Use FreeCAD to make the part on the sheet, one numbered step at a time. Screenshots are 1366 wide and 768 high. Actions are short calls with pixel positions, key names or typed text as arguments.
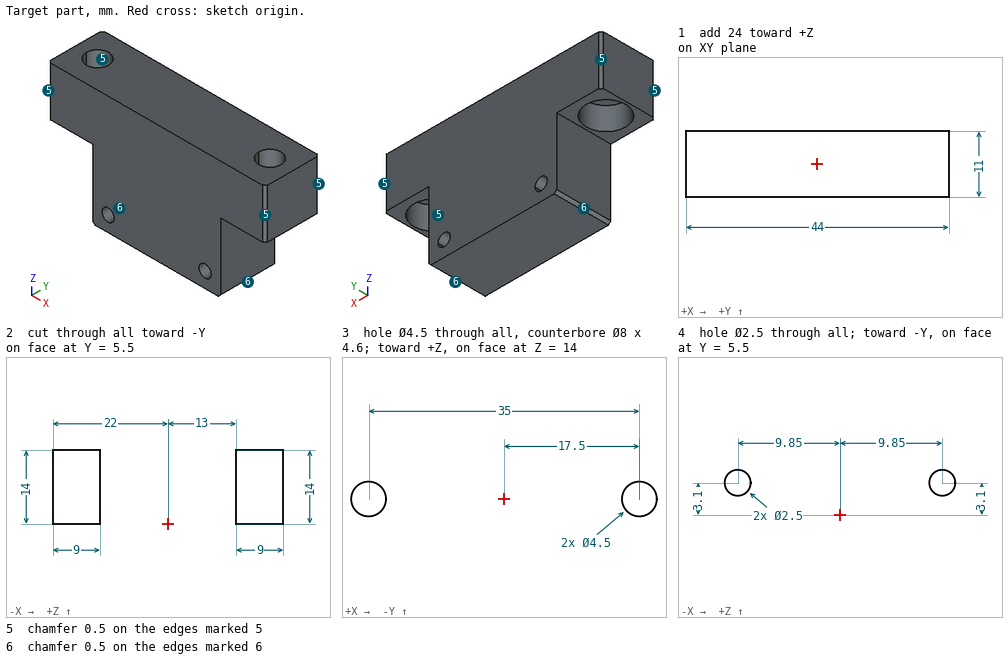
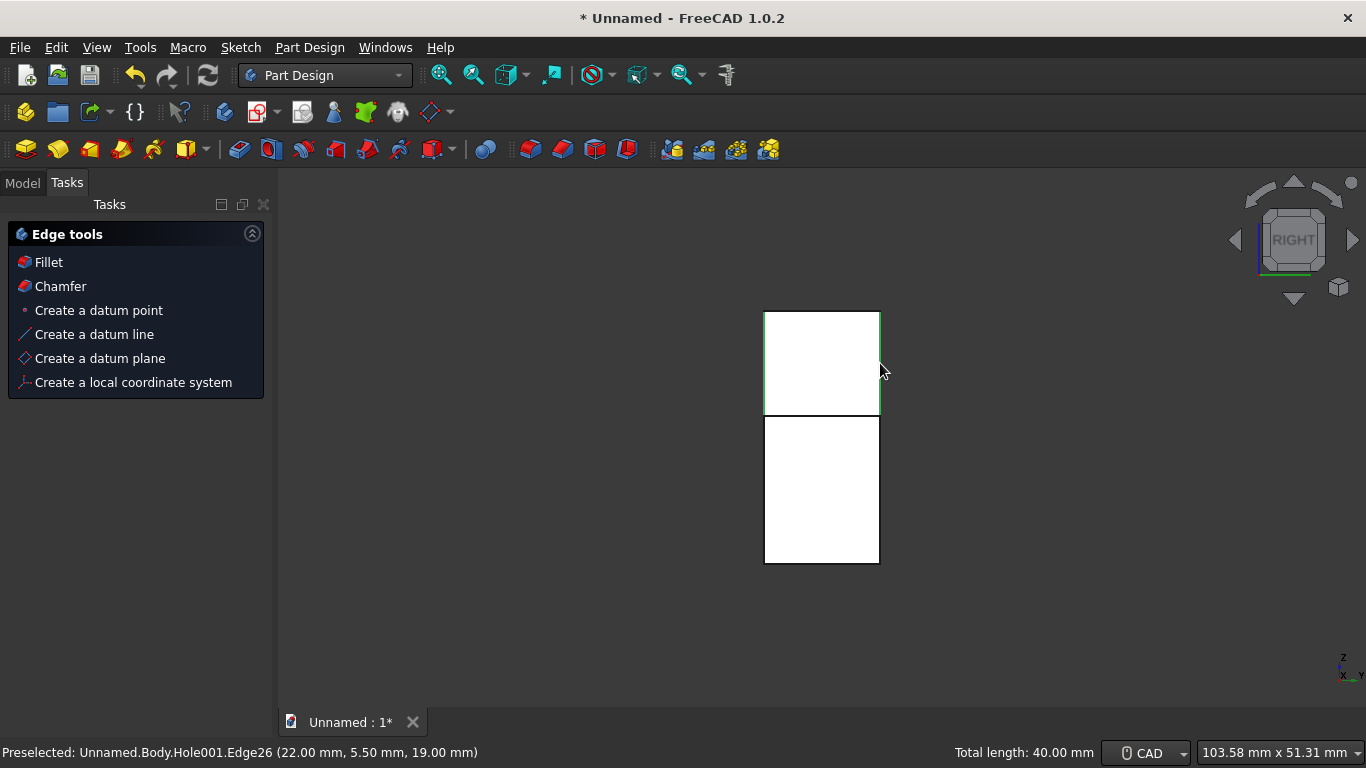
click(564, 150)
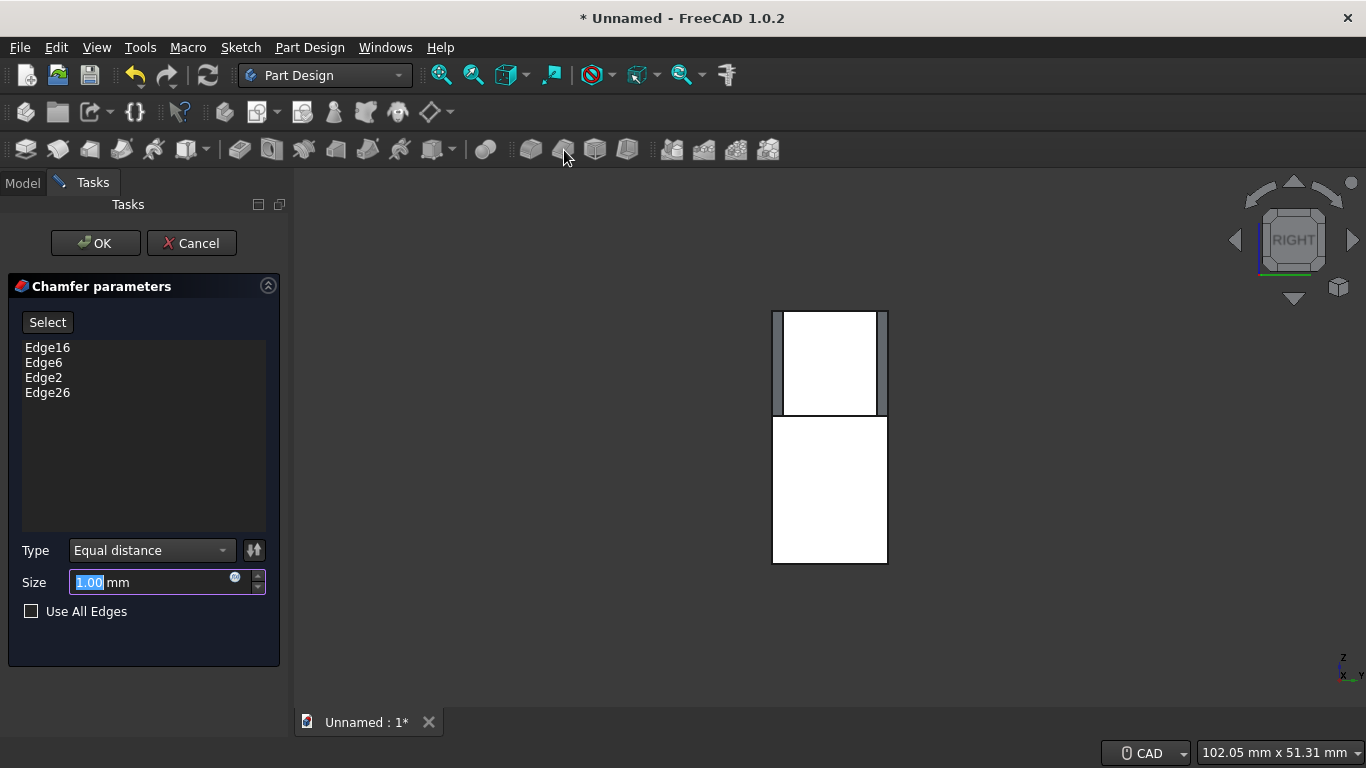
text(0.5)
key(Tab)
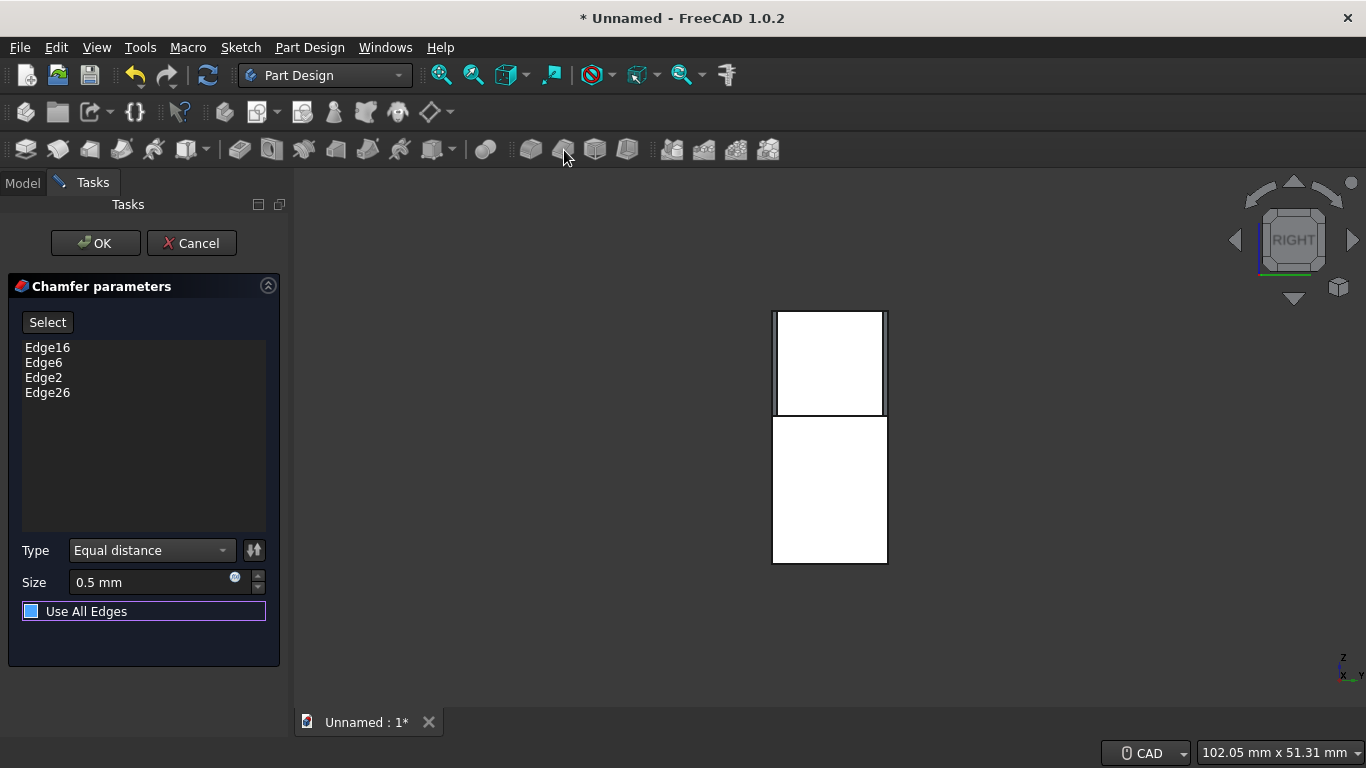
click(96, 243)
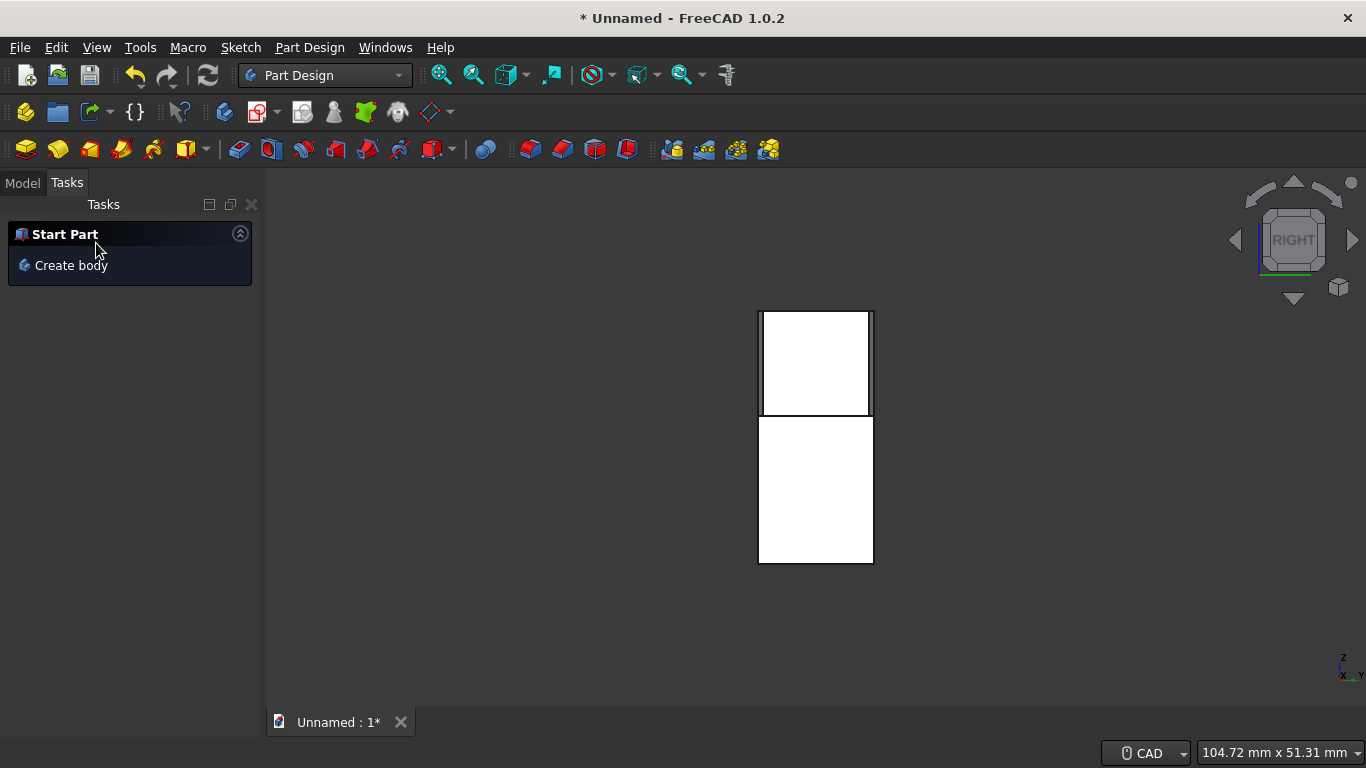
click(816, 563)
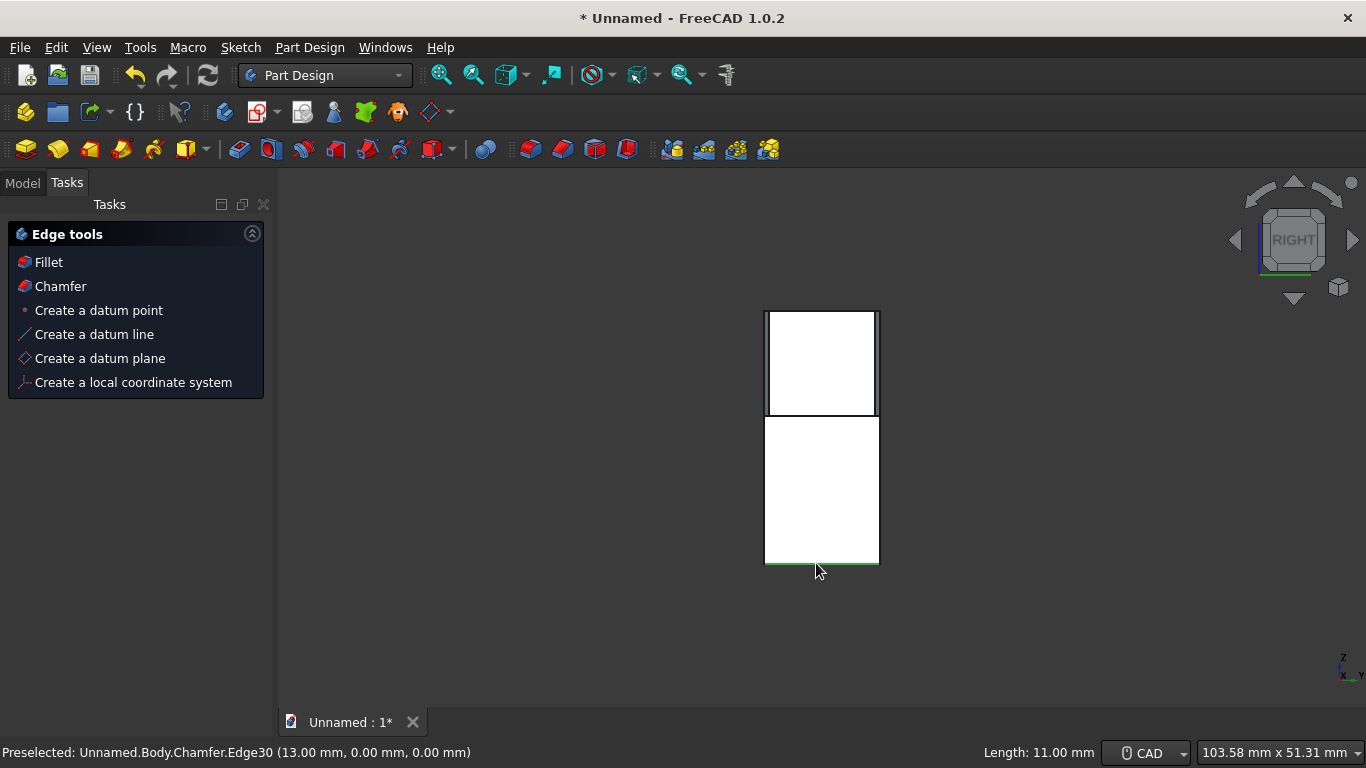
key(0)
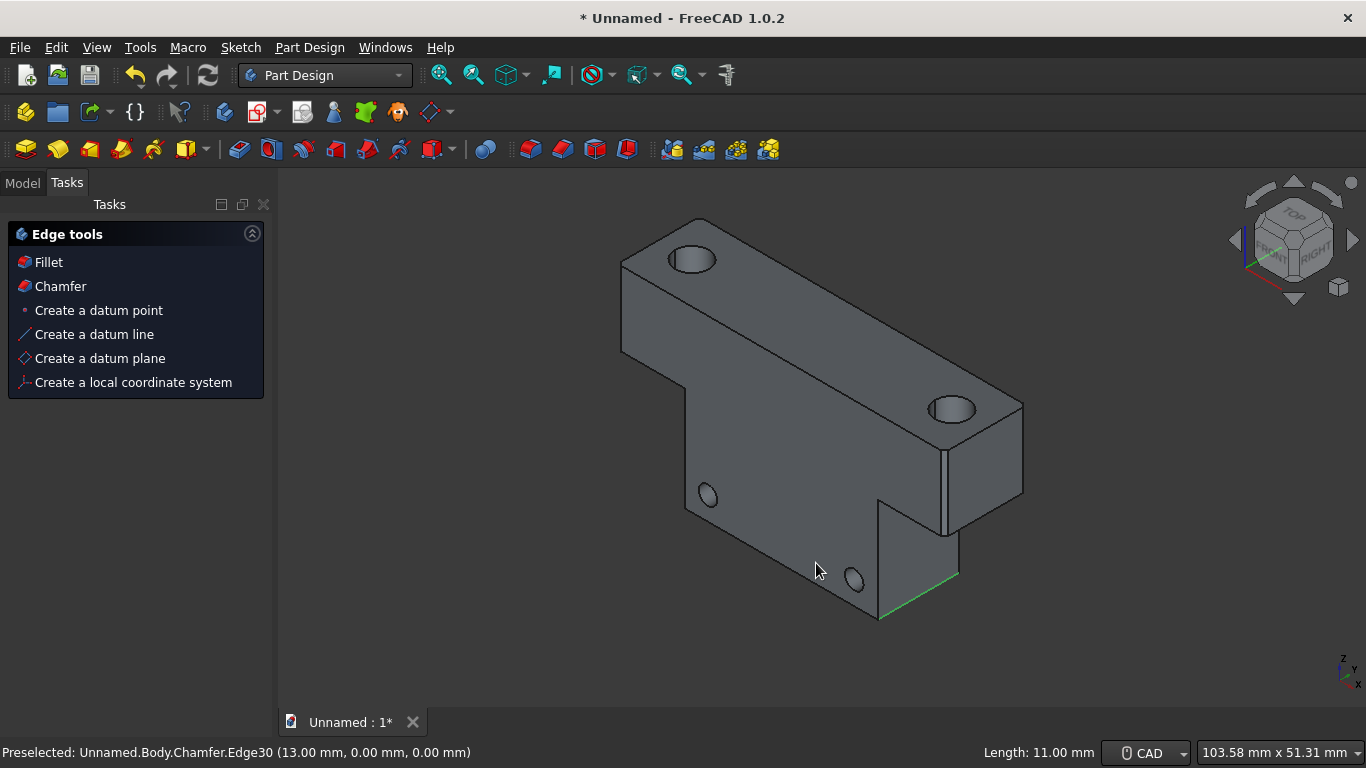
key(2)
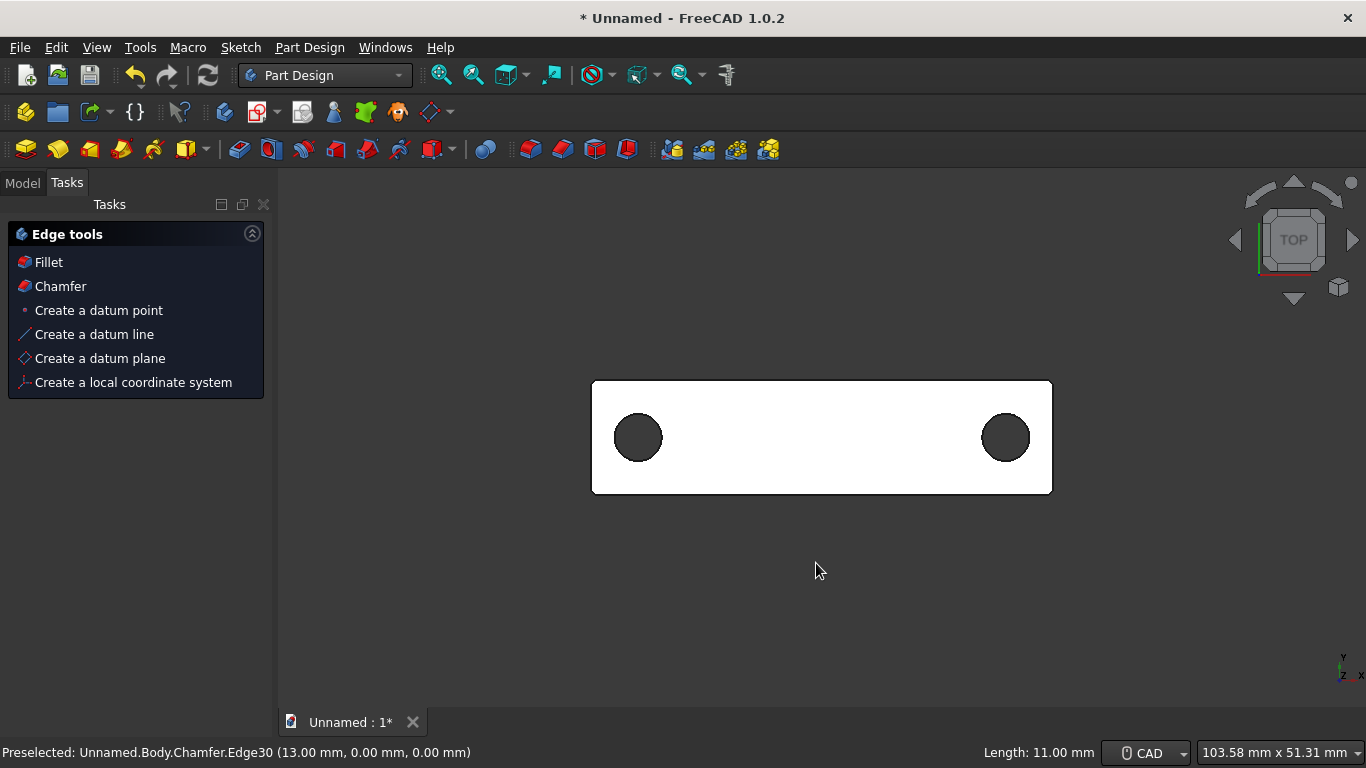
click(442, 76)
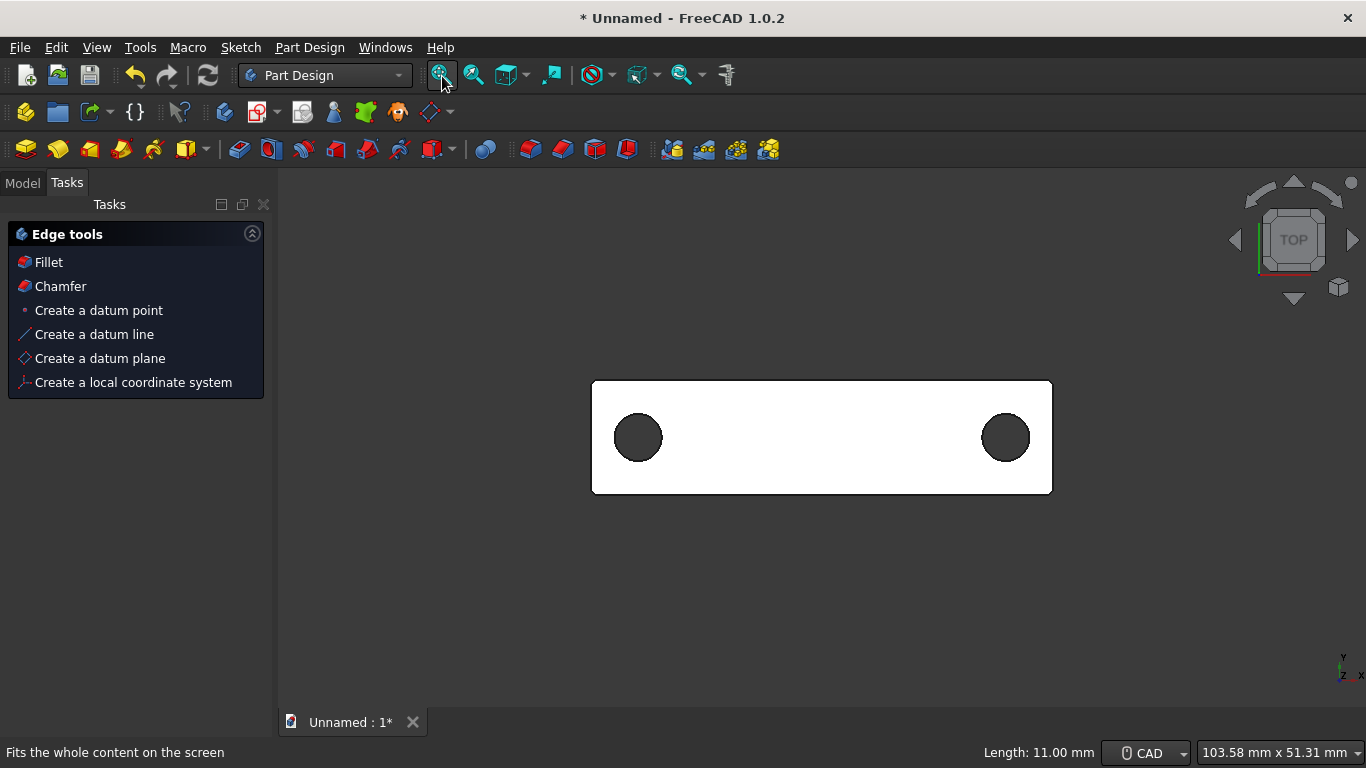
key(1)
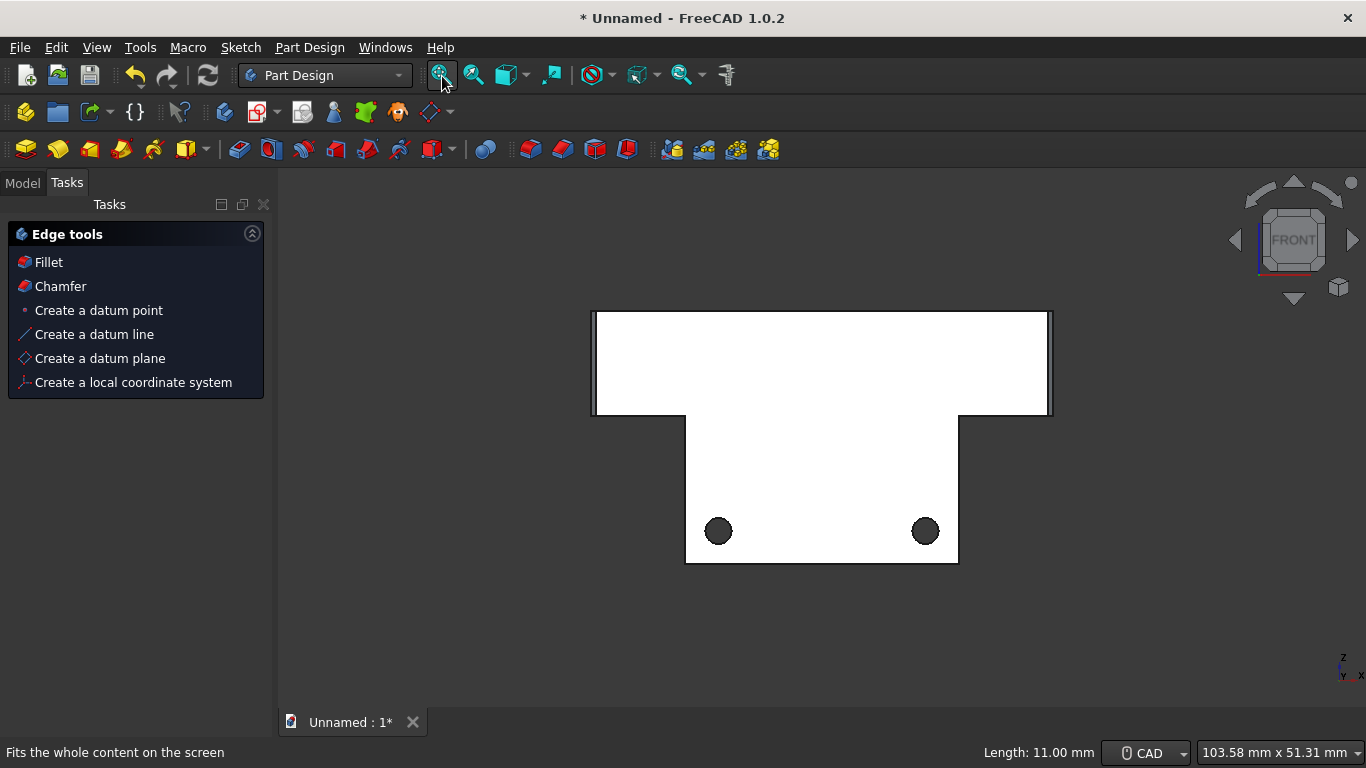
key(3)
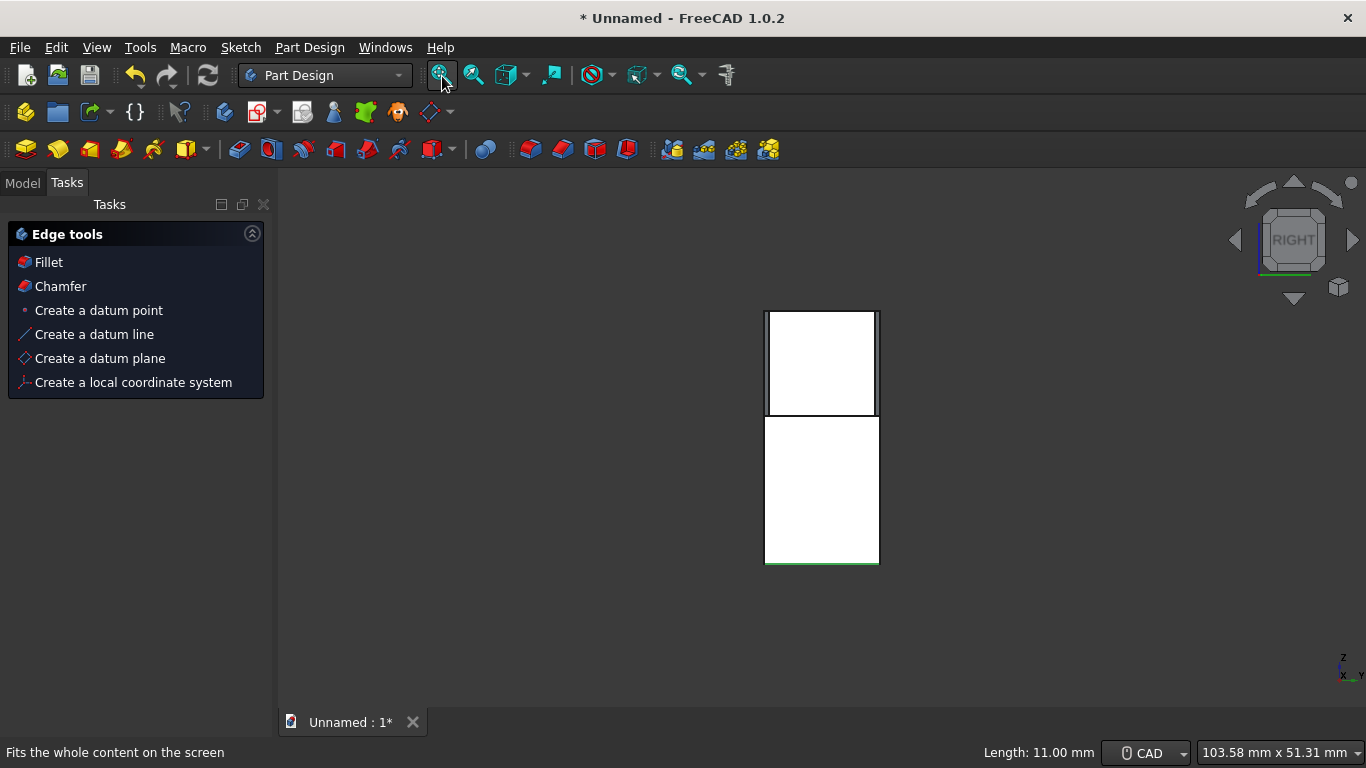
key(5)